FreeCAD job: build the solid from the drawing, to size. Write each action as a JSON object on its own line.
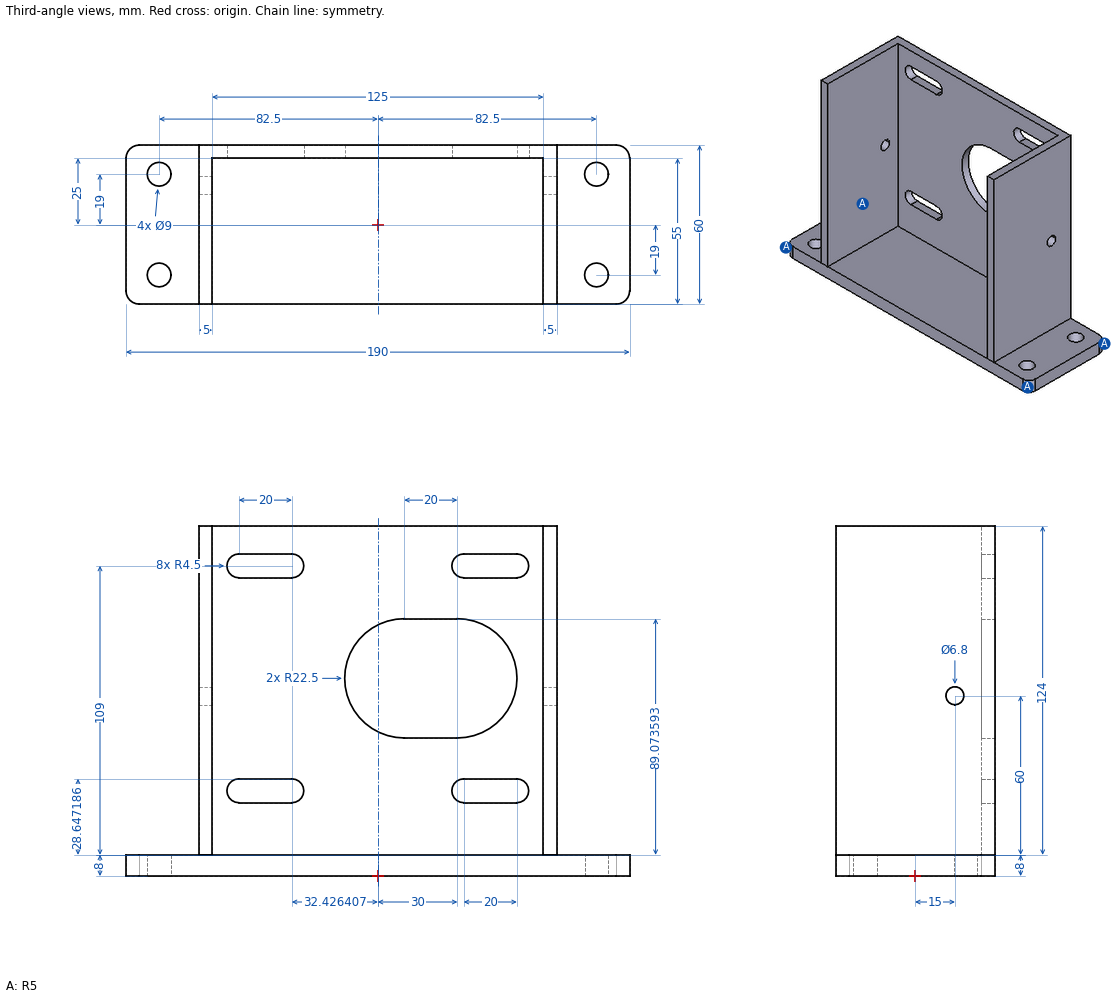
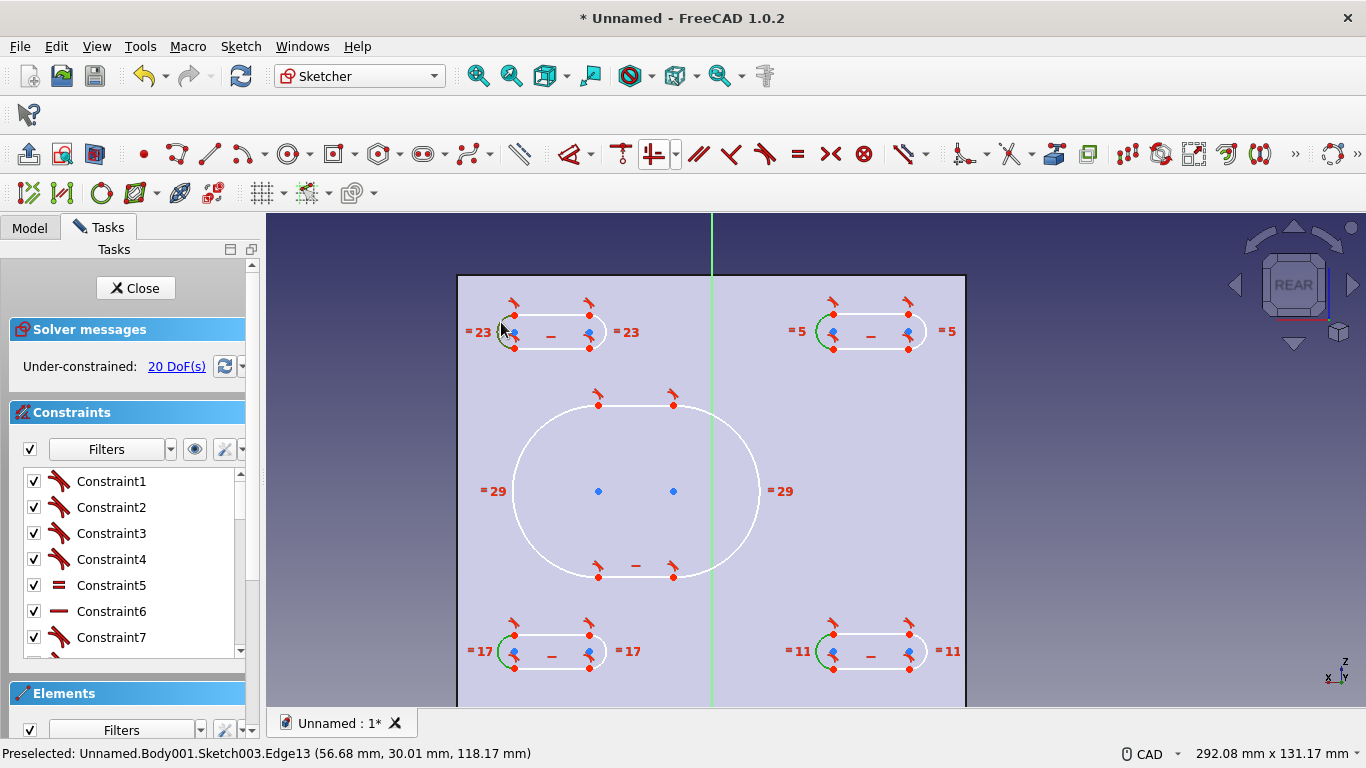
{"action": "left_click", "coordinate": [798, 154]}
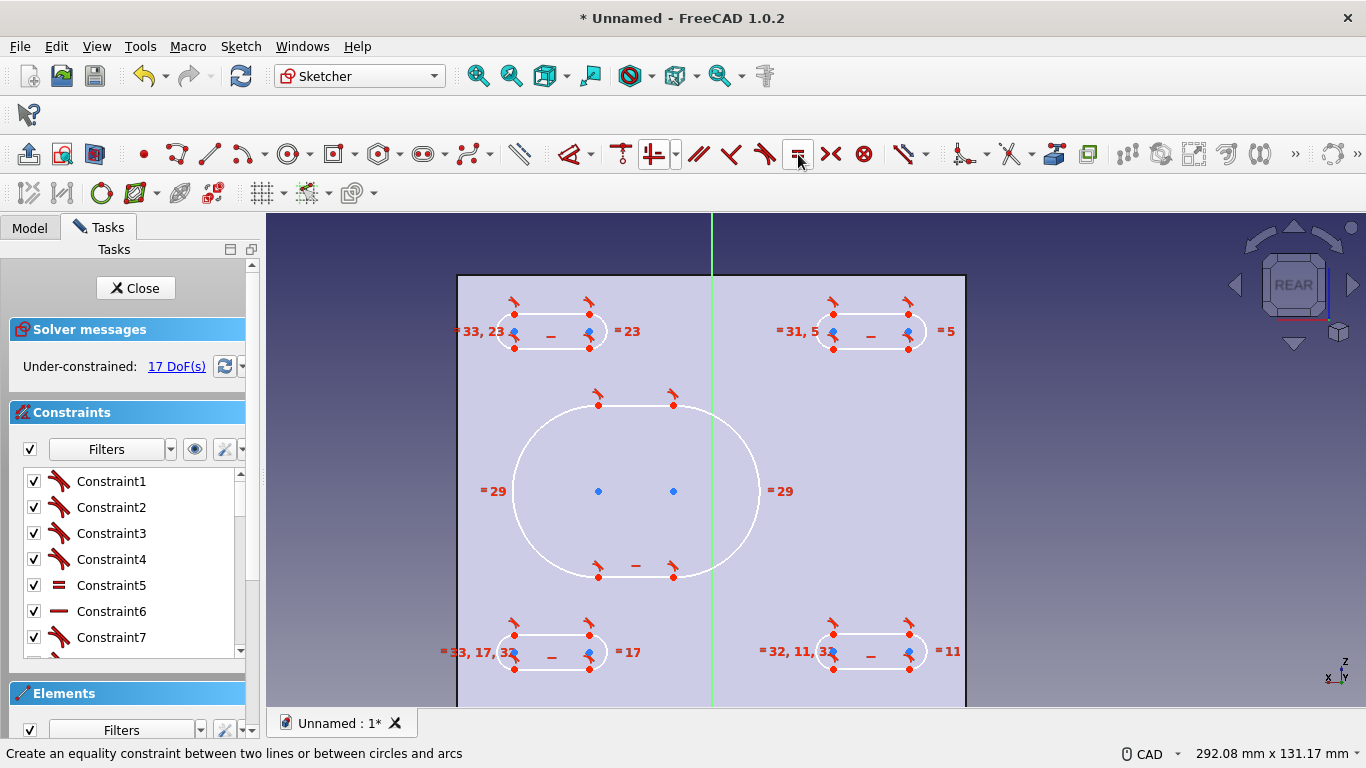
{"action": "left_click", "coordinate": [909, 652]}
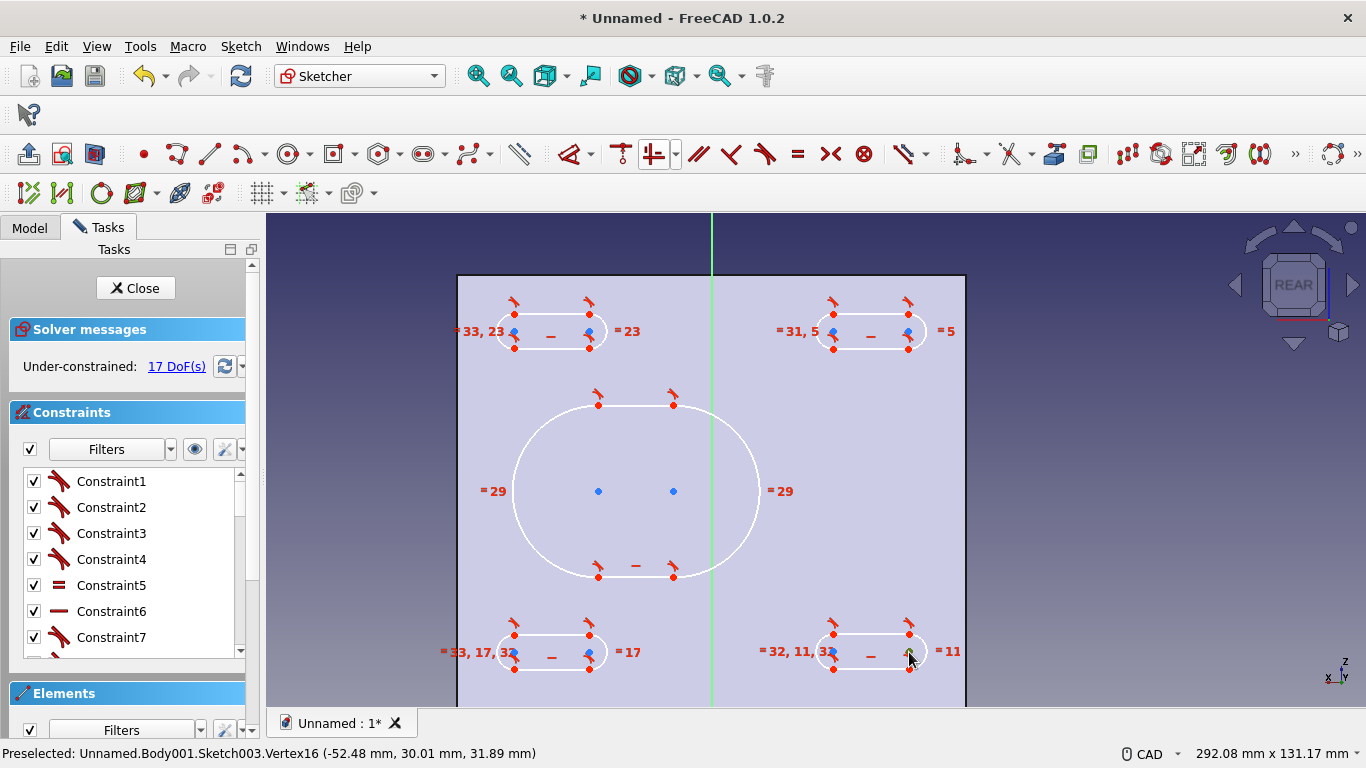
{"action": "left_click", "coordinate": [515, 652]}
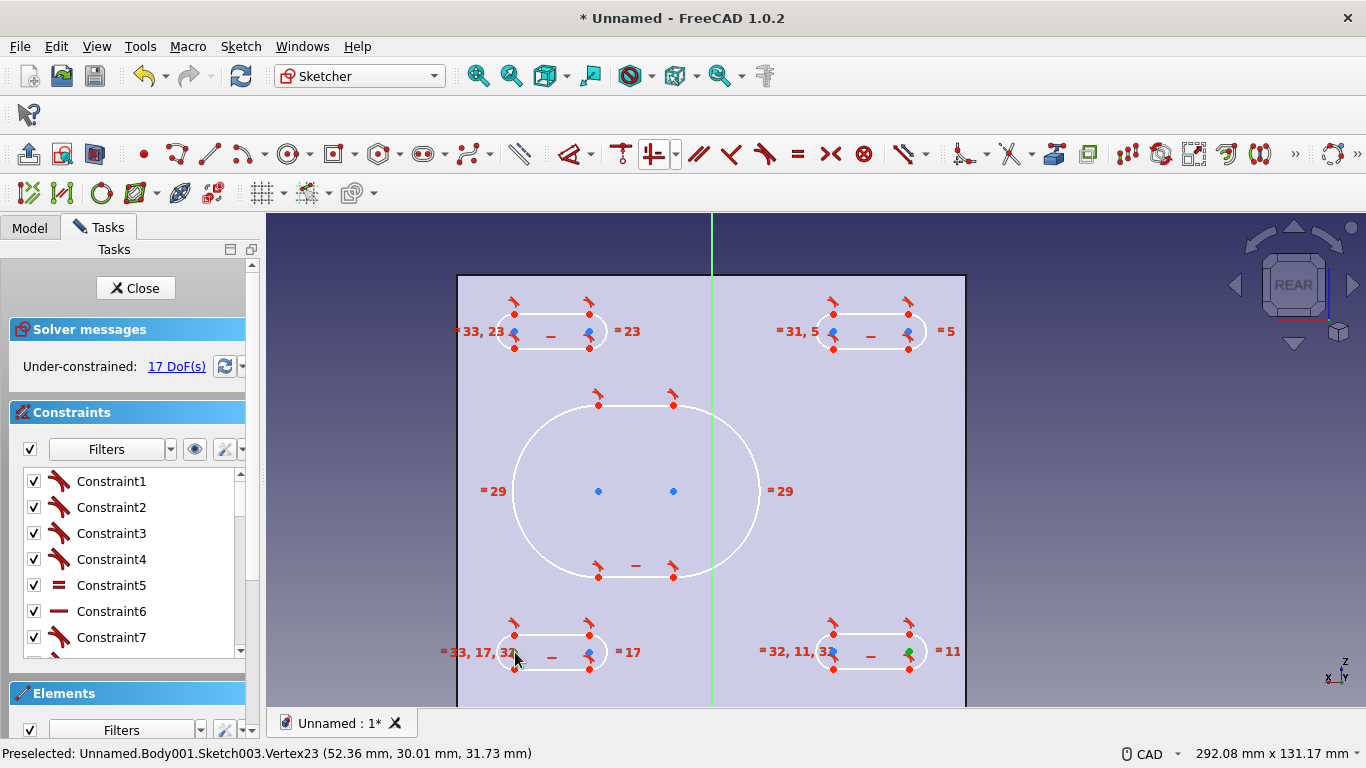
{"action": "left_click", "coordinate": [712, 648]}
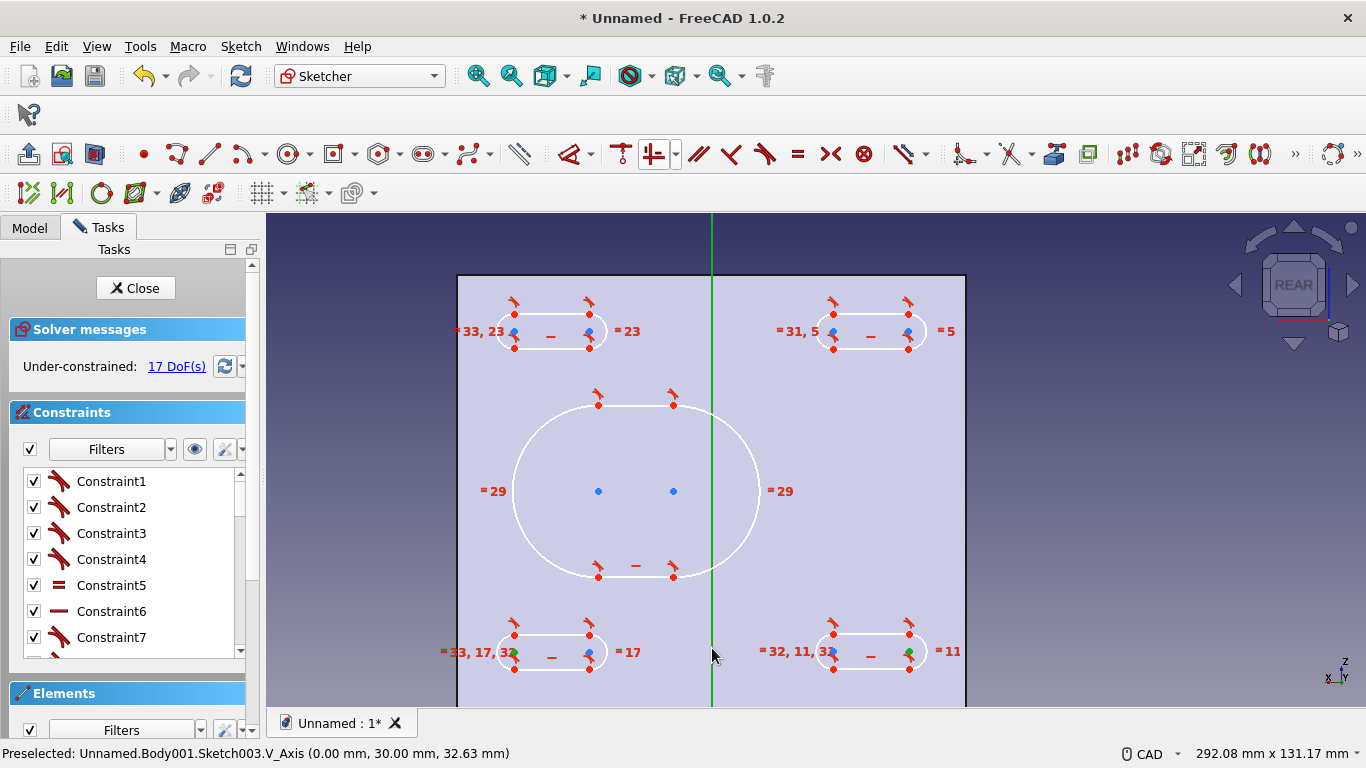
{"action": "left_click", "coordinate": [831, 154]}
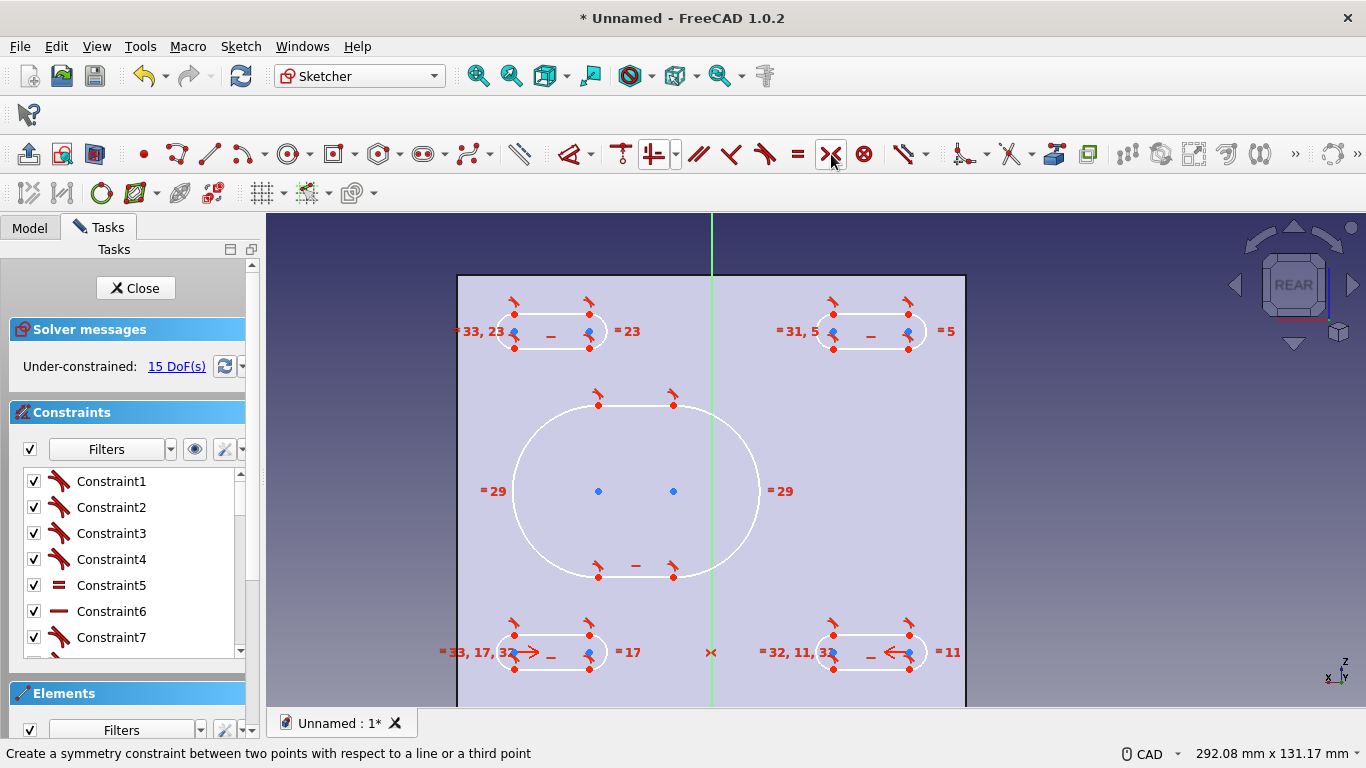
{"action": "left_click", "coordinate": [909, 332]}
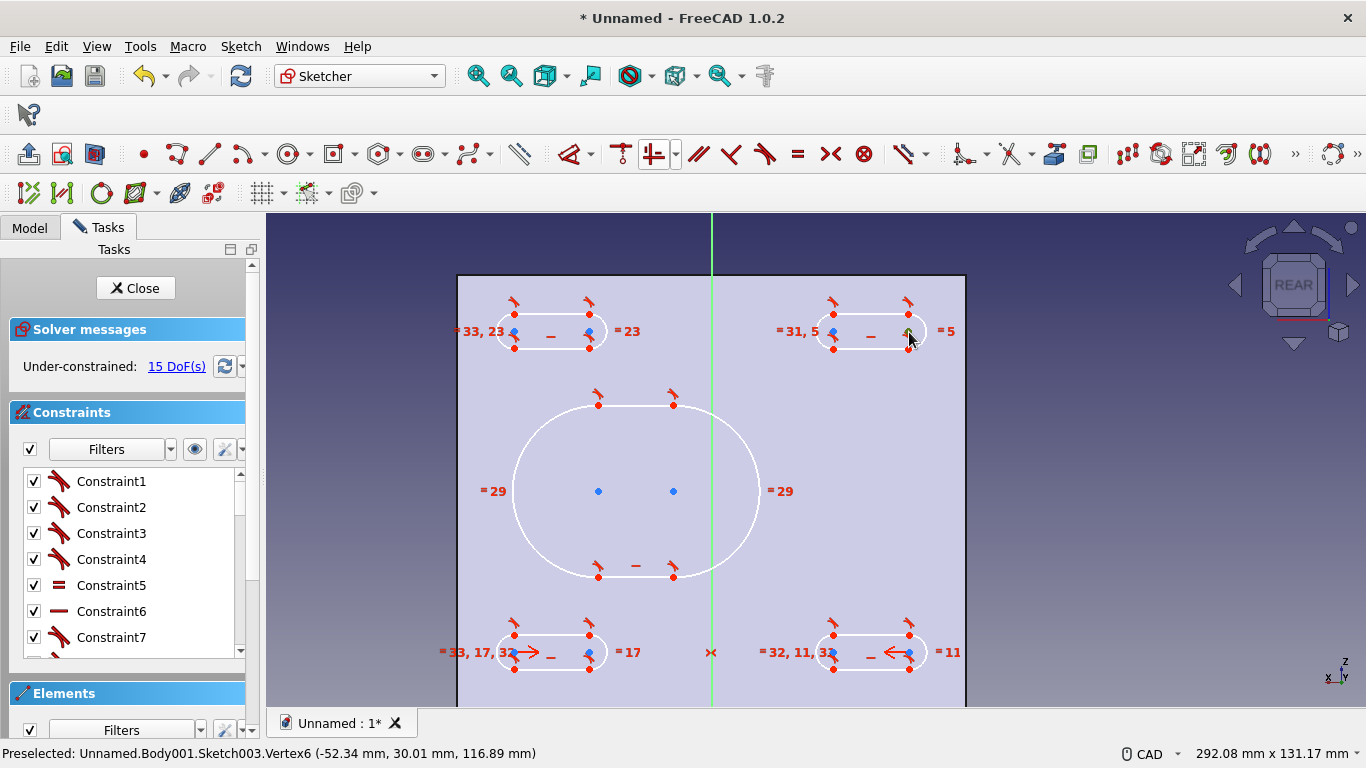
{"action": "left_click", "coordinate": [514, 331]}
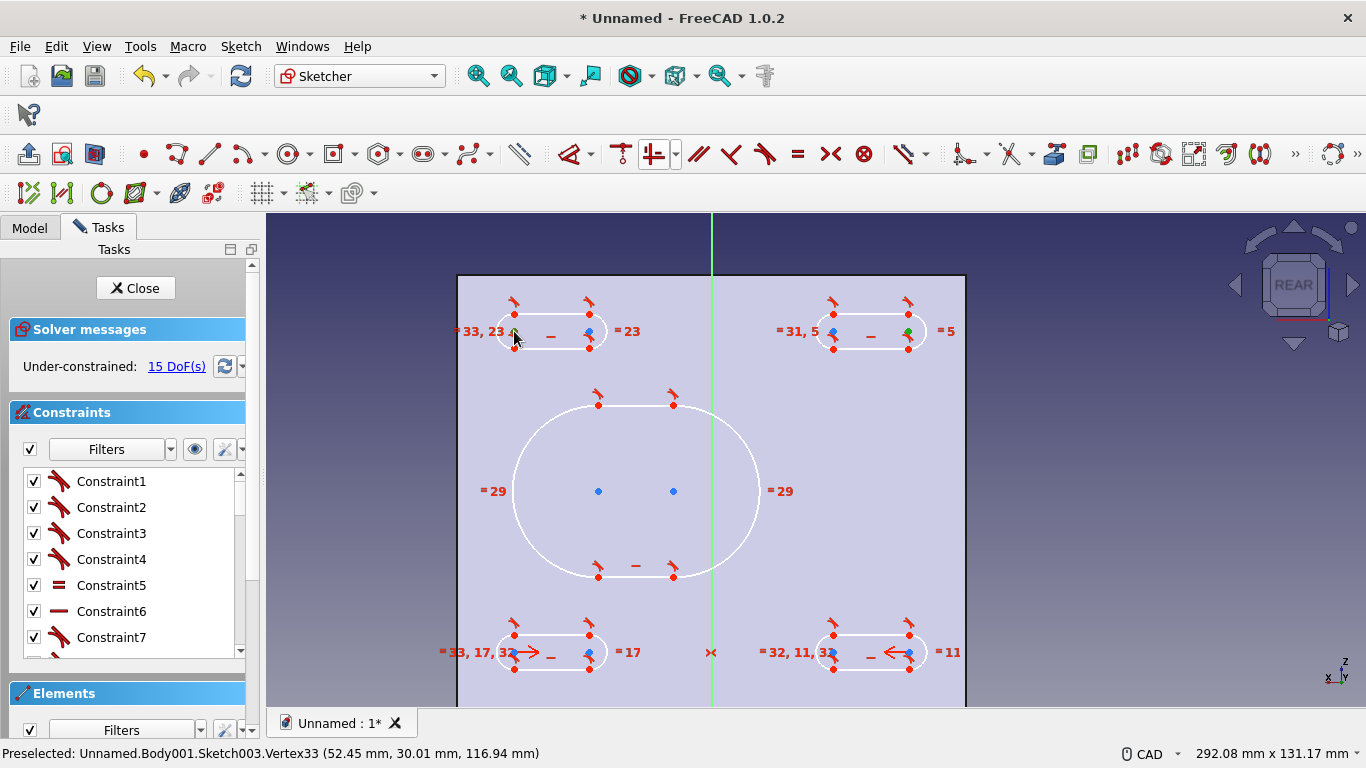
{"action": "left_click", "coordinate": [712, 616]}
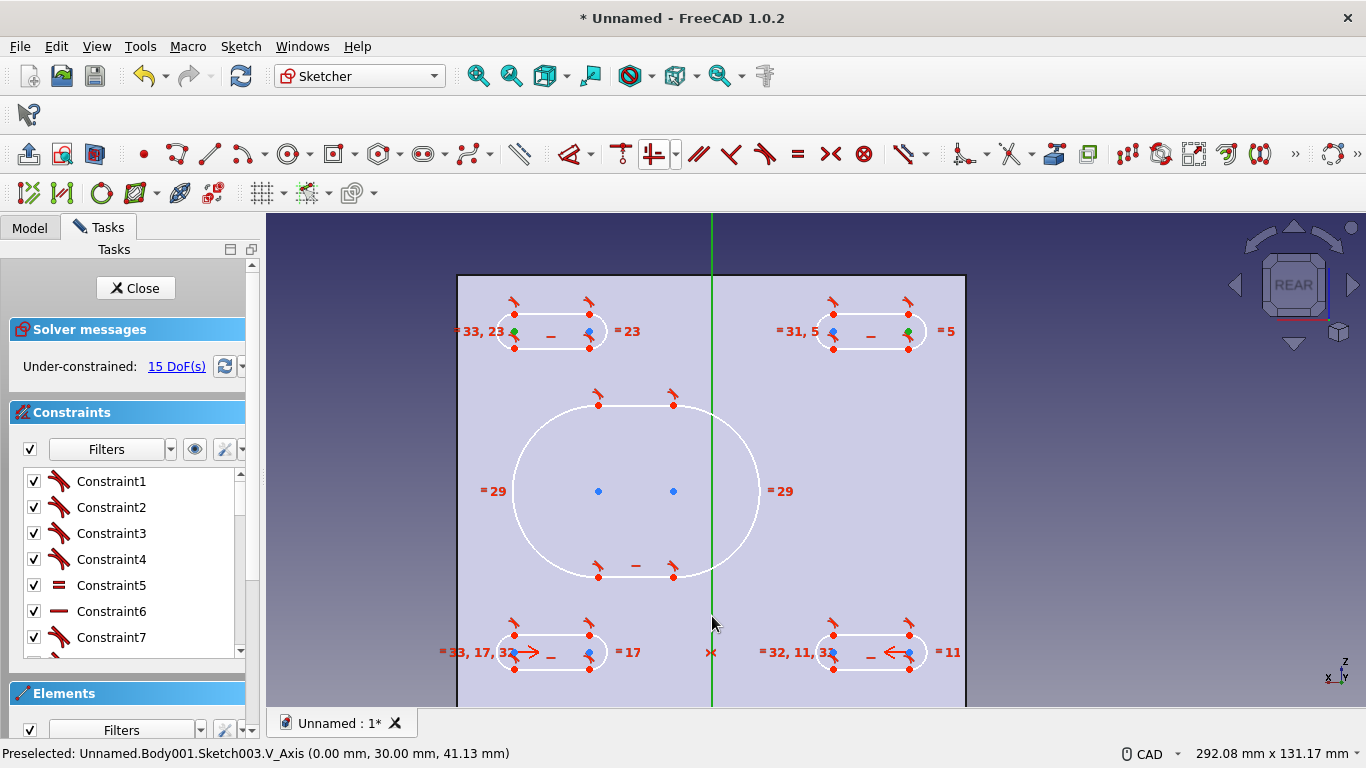
{"action": "left_click", "coordinate": [831, 154]}